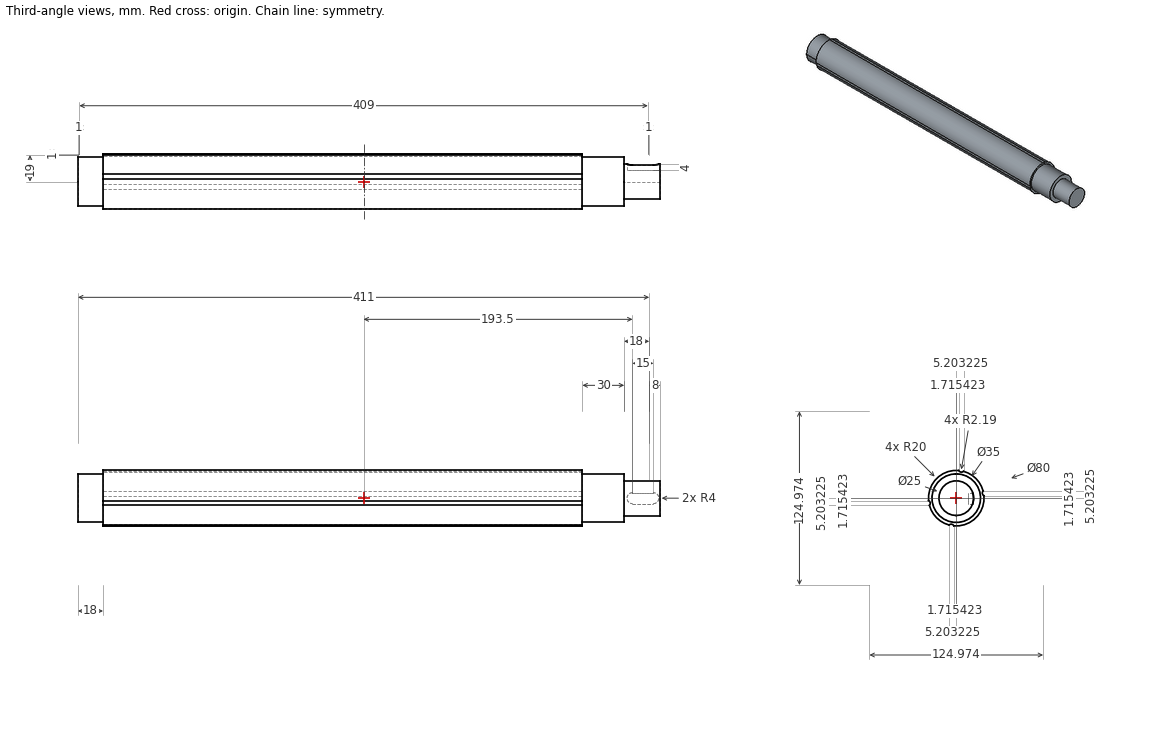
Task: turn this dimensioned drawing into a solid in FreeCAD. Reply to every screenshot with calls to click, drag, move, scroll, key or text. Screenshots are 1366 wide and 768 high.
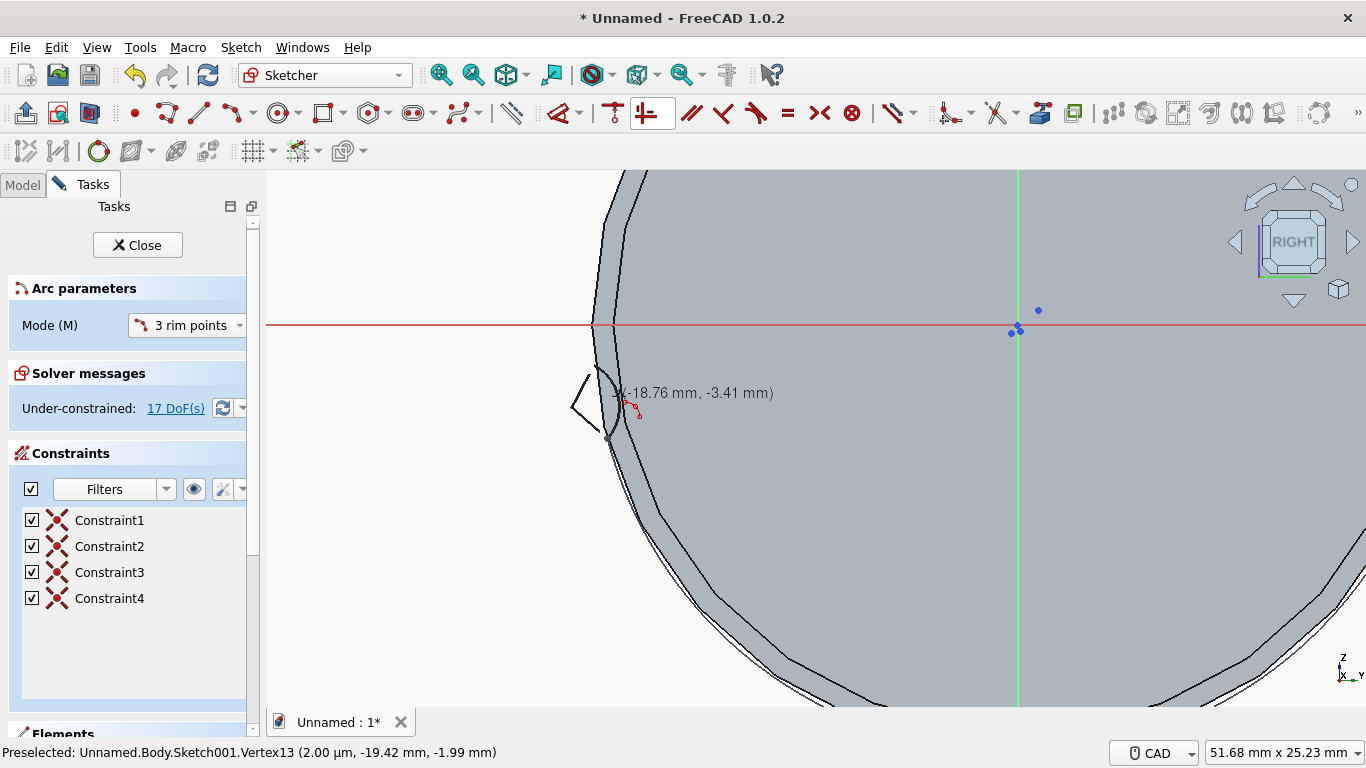
click(619, 396)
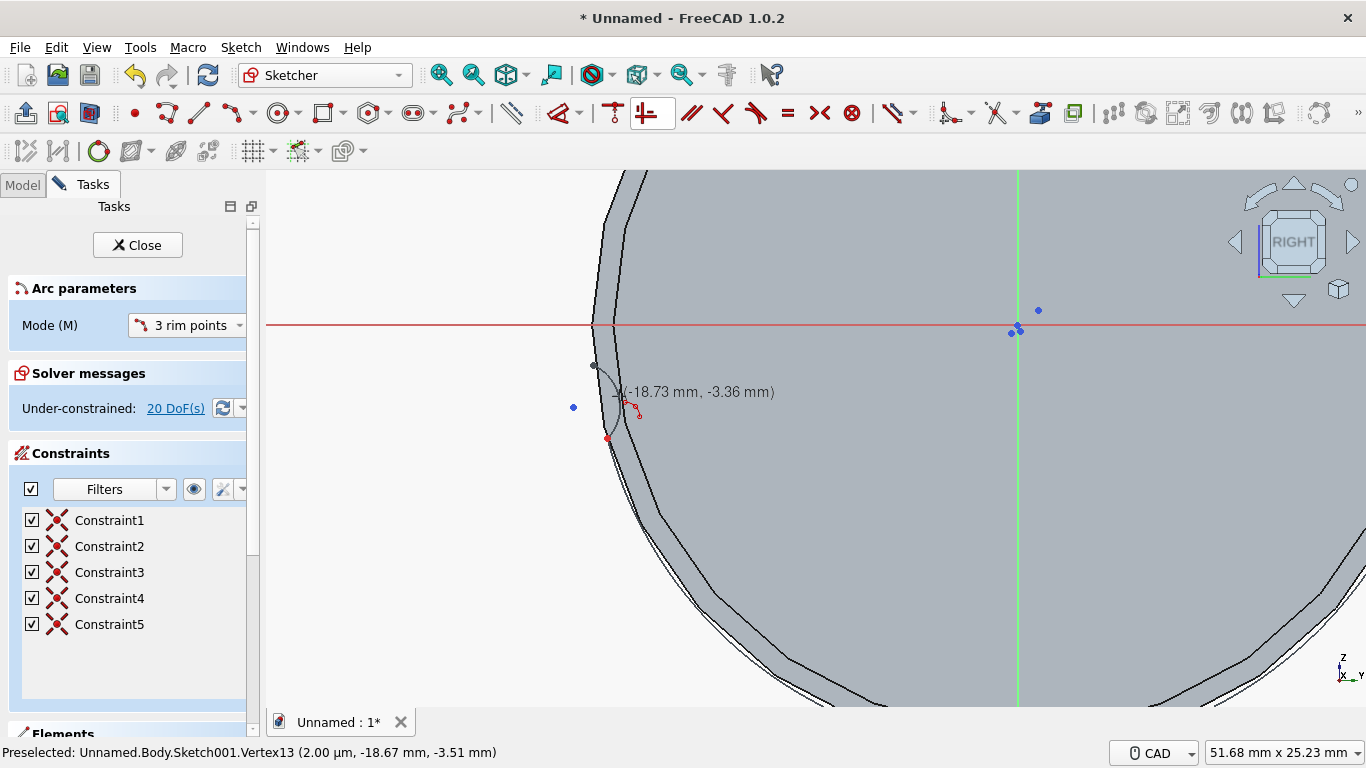
click(594, 365)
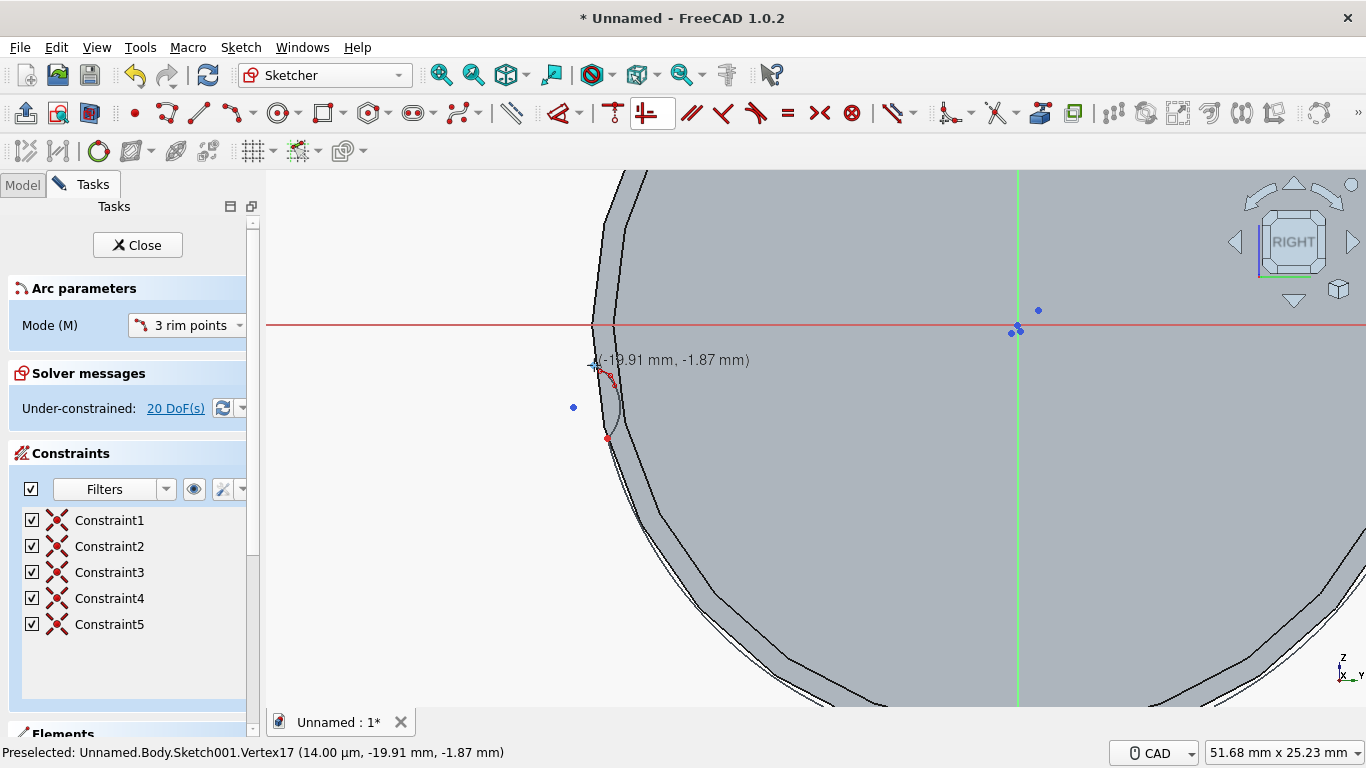
scroll(679, 467, down, 8)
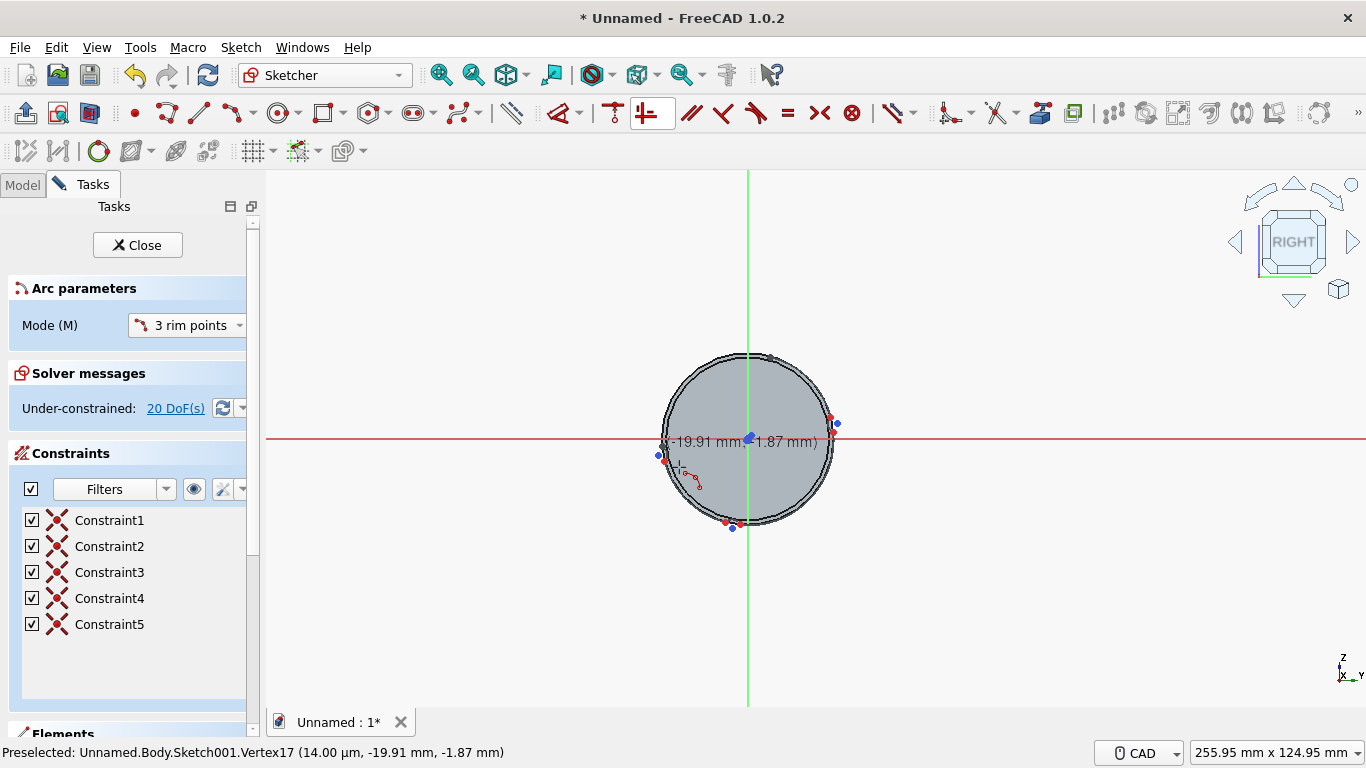
scroll(755, 353, up, 4)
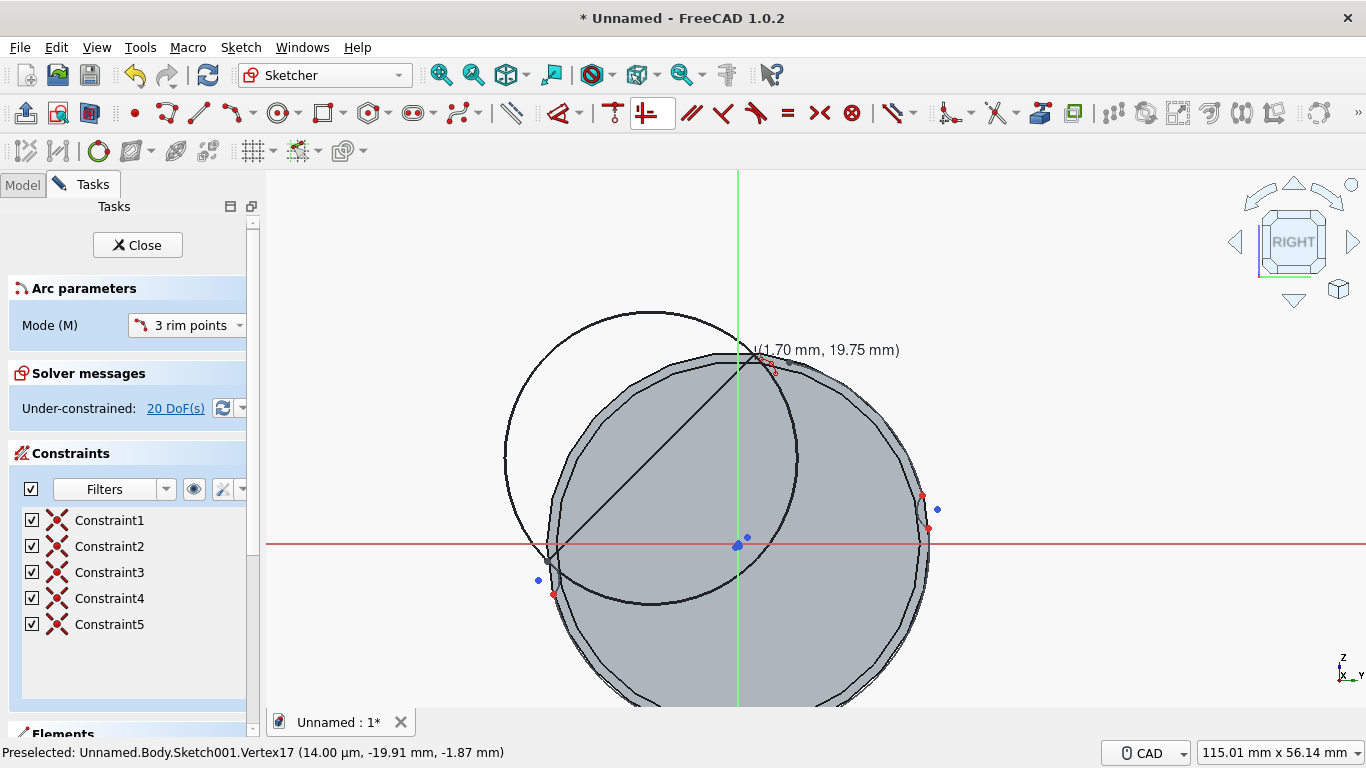
click(755, 353)
click(603, 408)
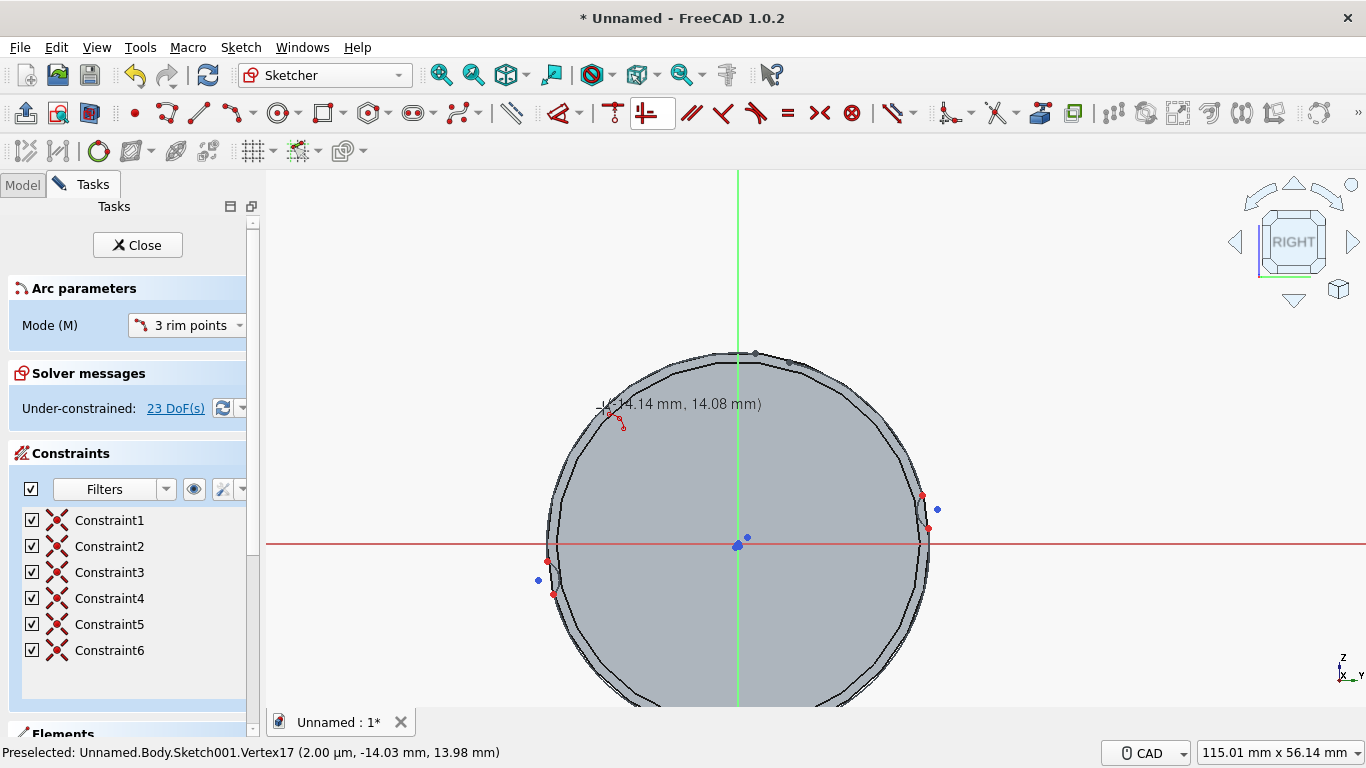
click(755, 354)
click(789, 362)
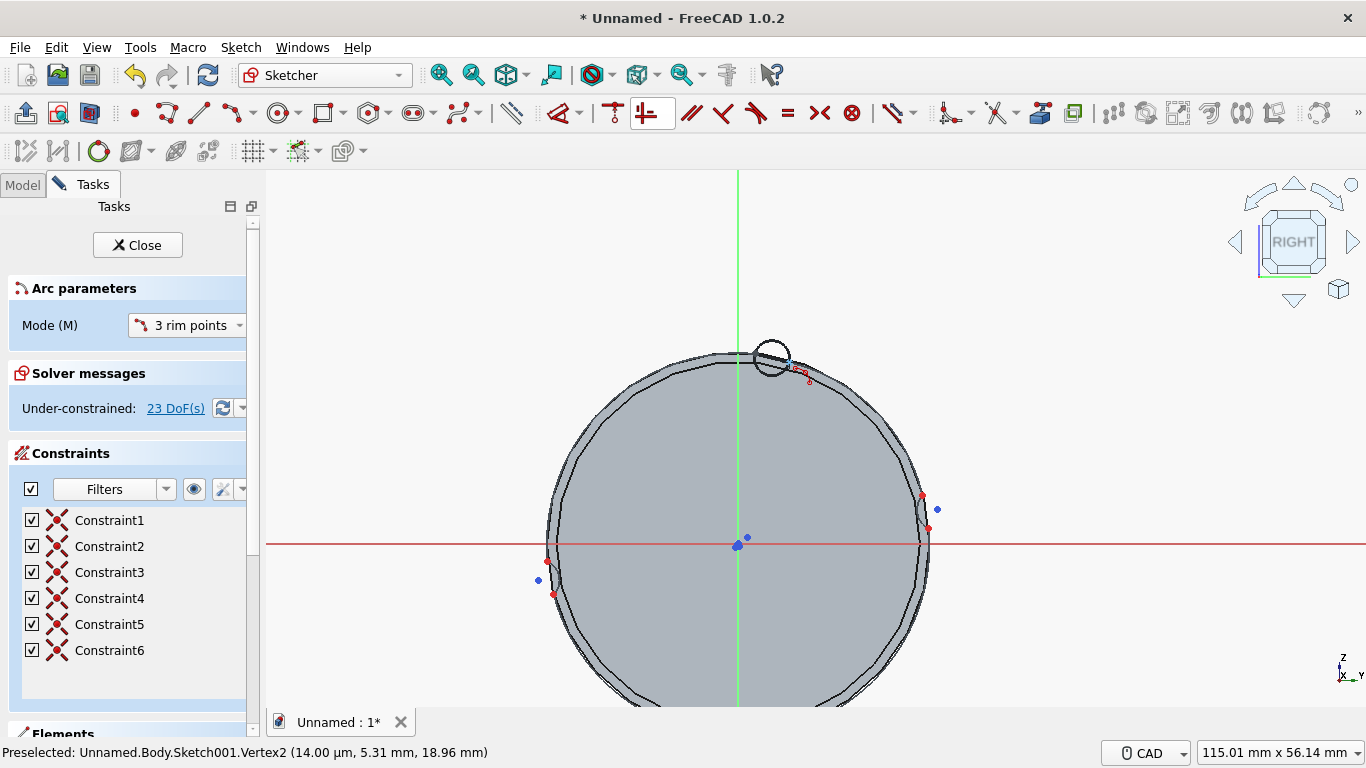
scroll(770, 365, up, 4)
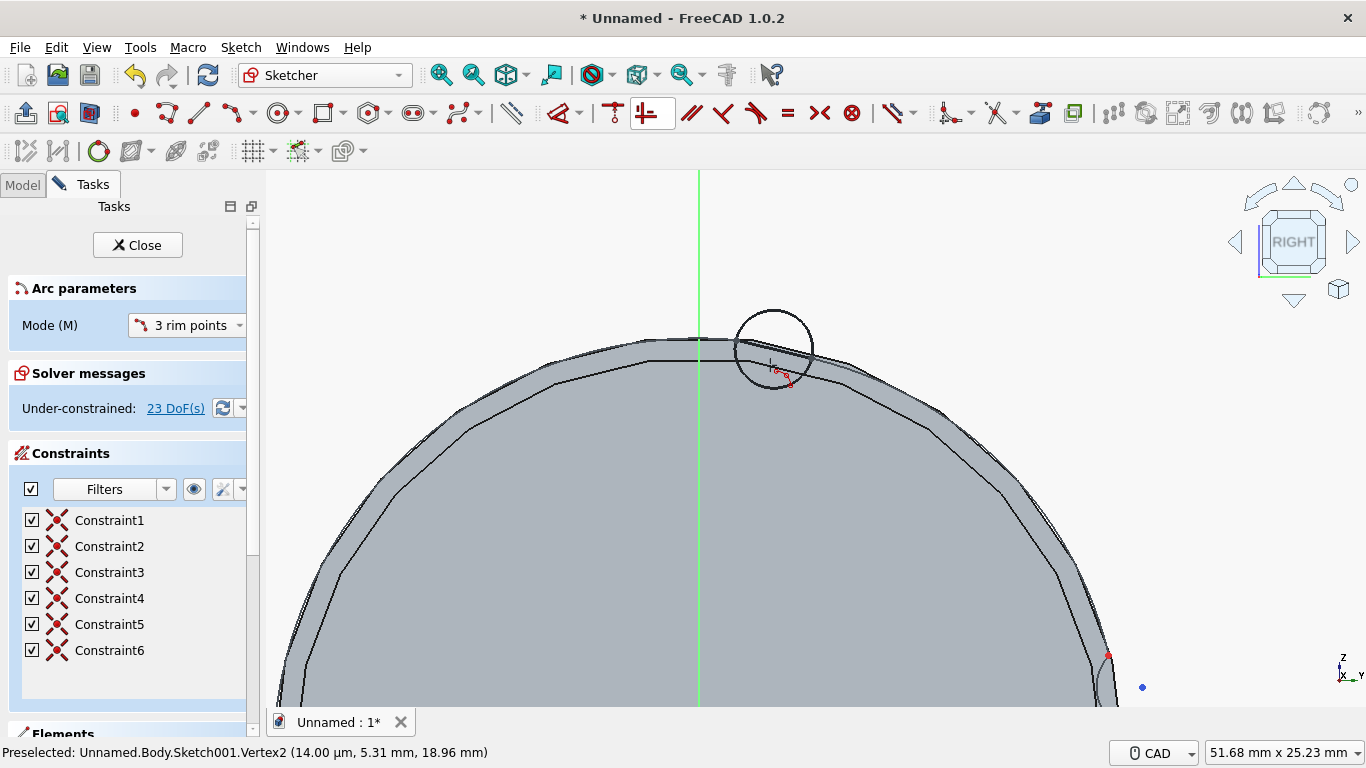
click(769, 364)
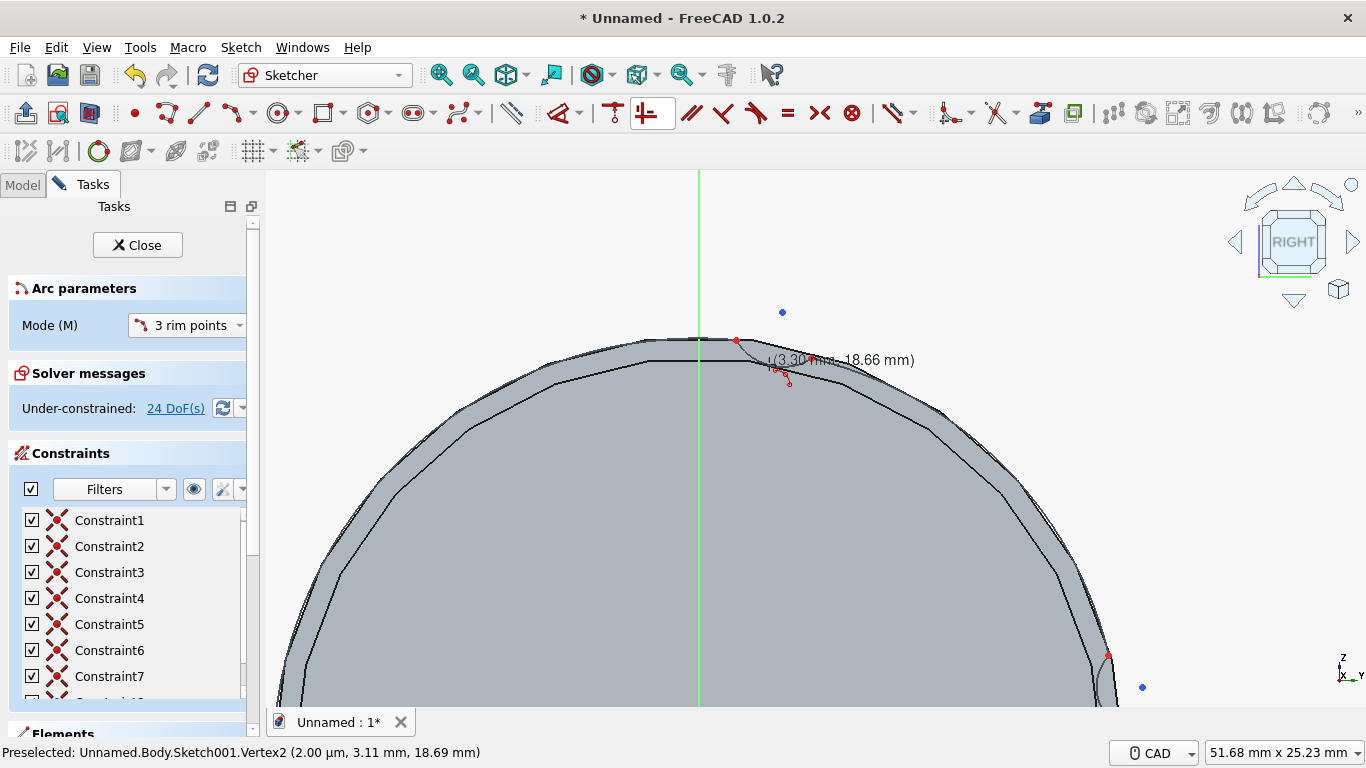
key(g)
key(c)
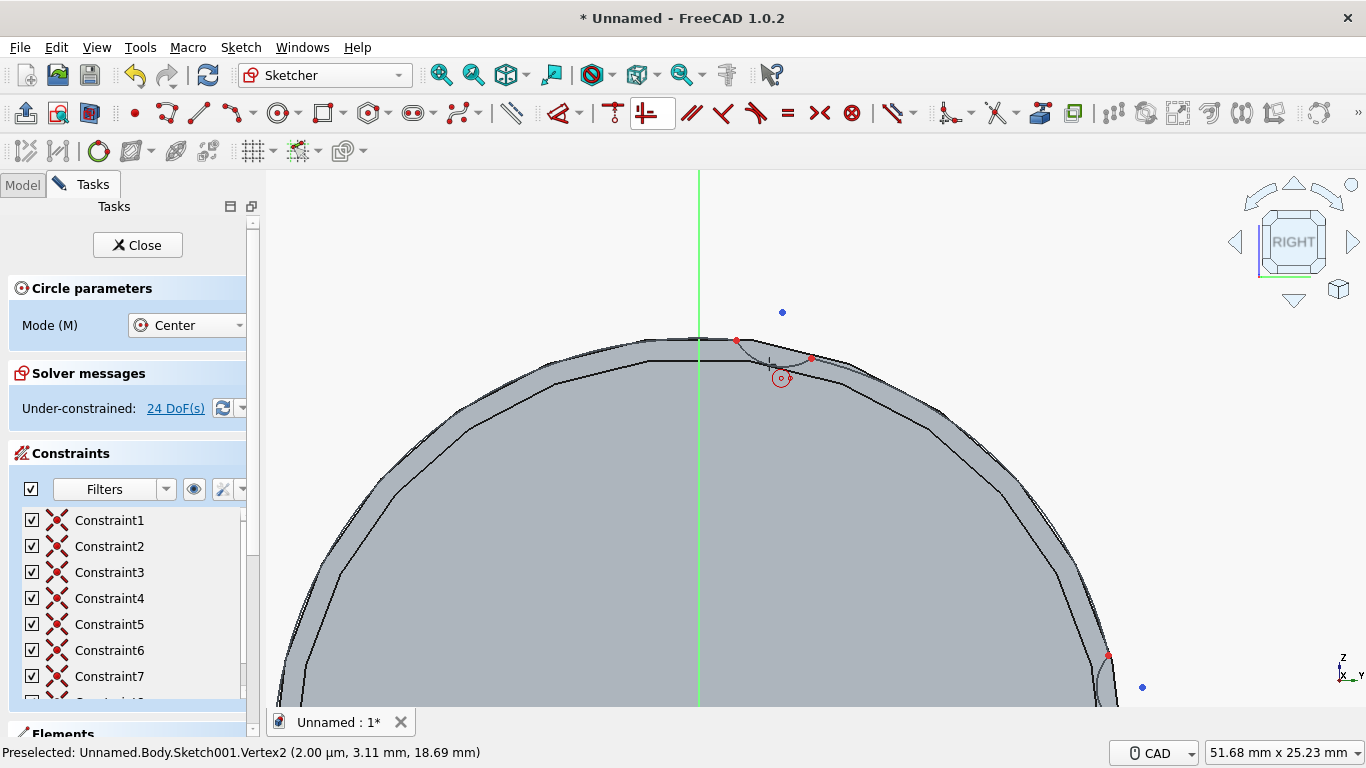
scroll(760, 357, down, 8)